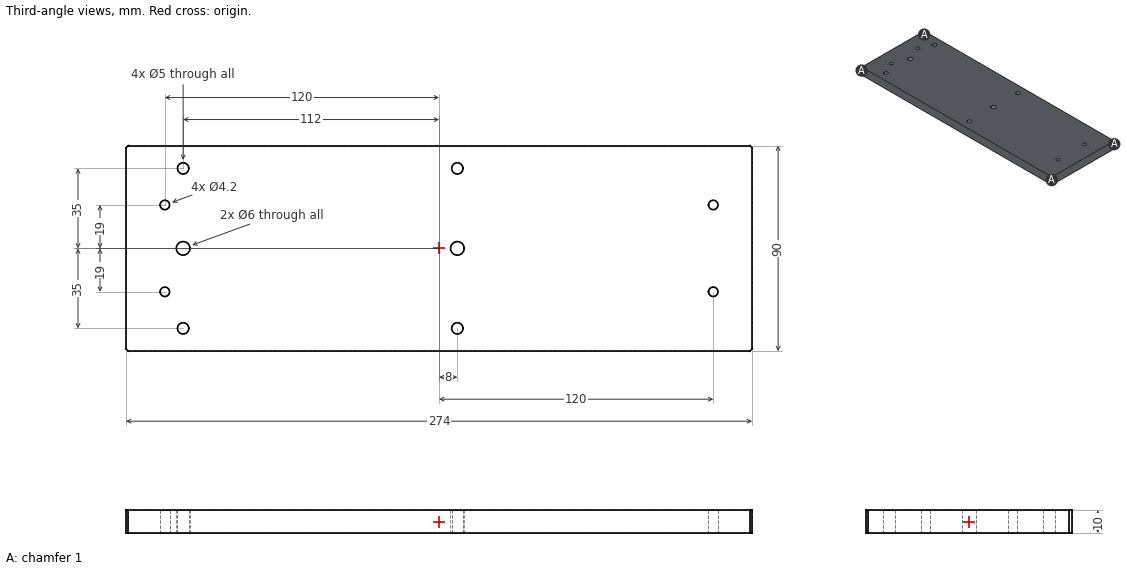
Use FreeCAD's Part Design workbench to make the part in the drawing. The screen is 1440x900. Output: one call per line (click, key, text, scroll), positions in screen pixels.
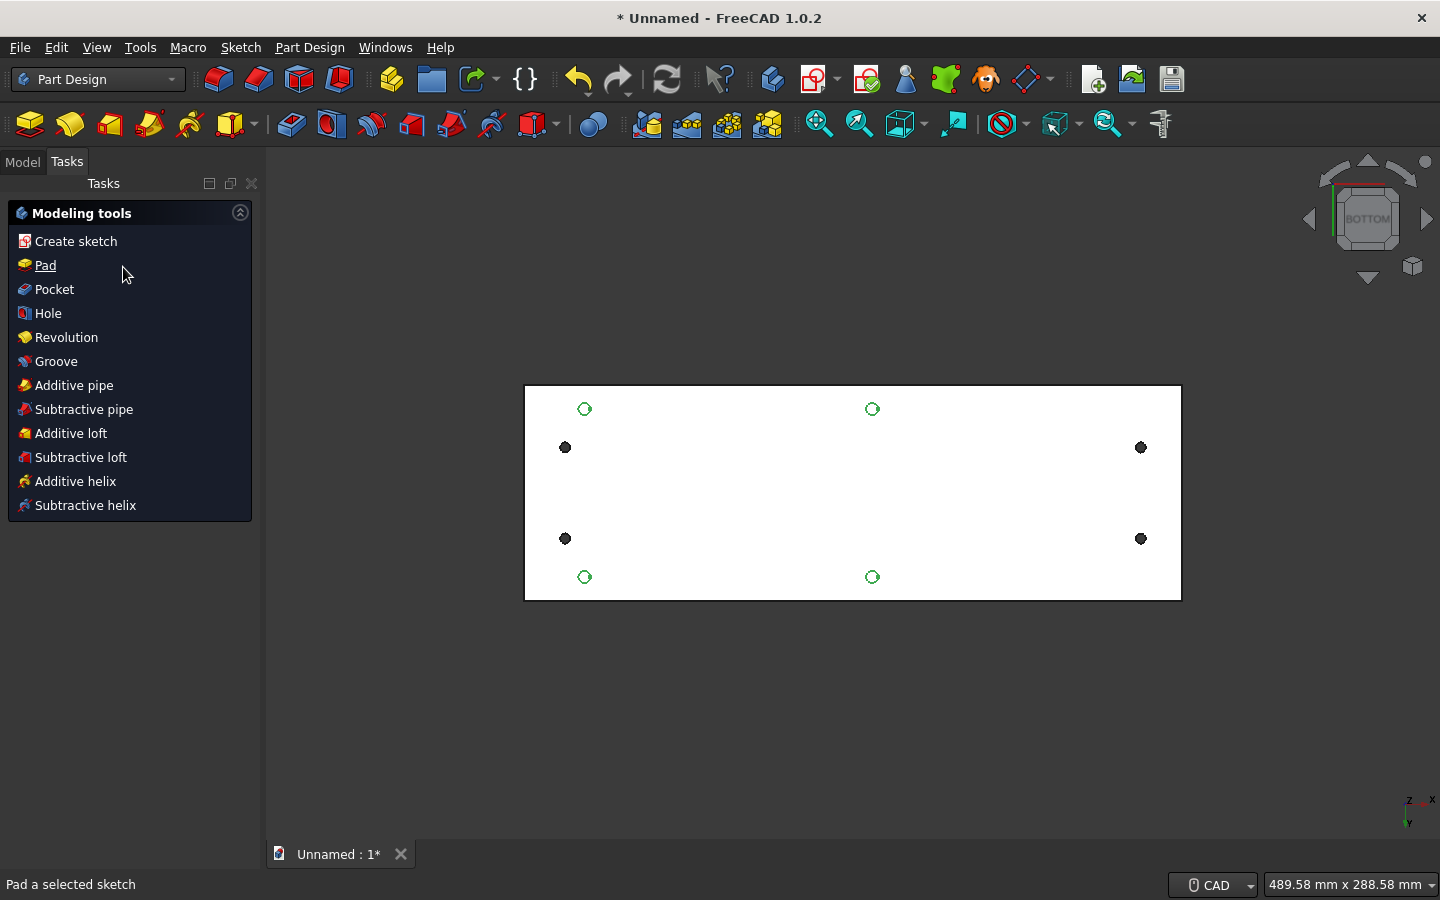
click(332, 124)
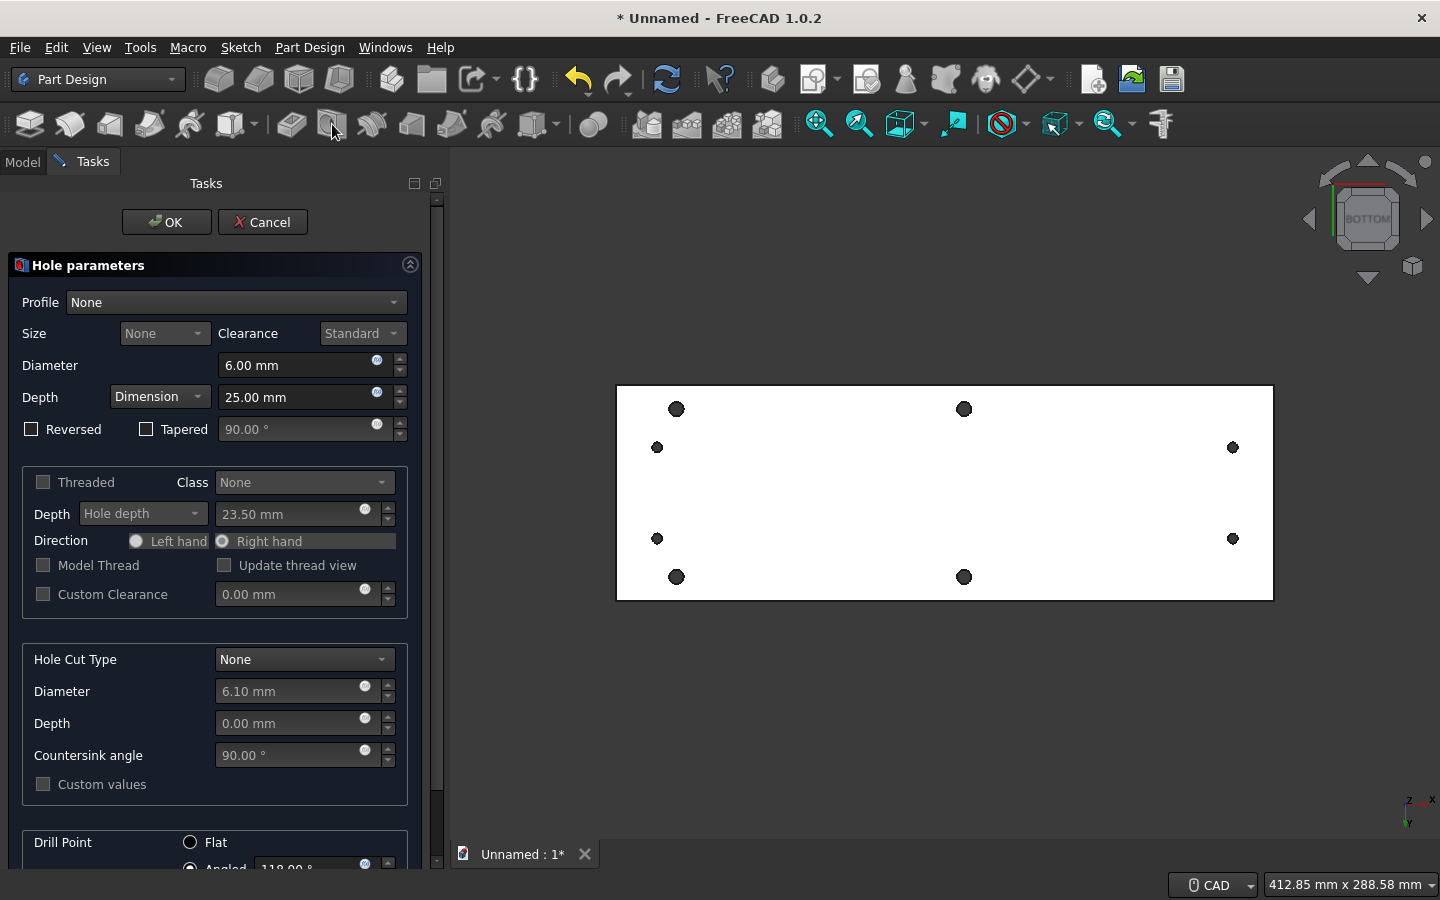
triple_click(305, 365)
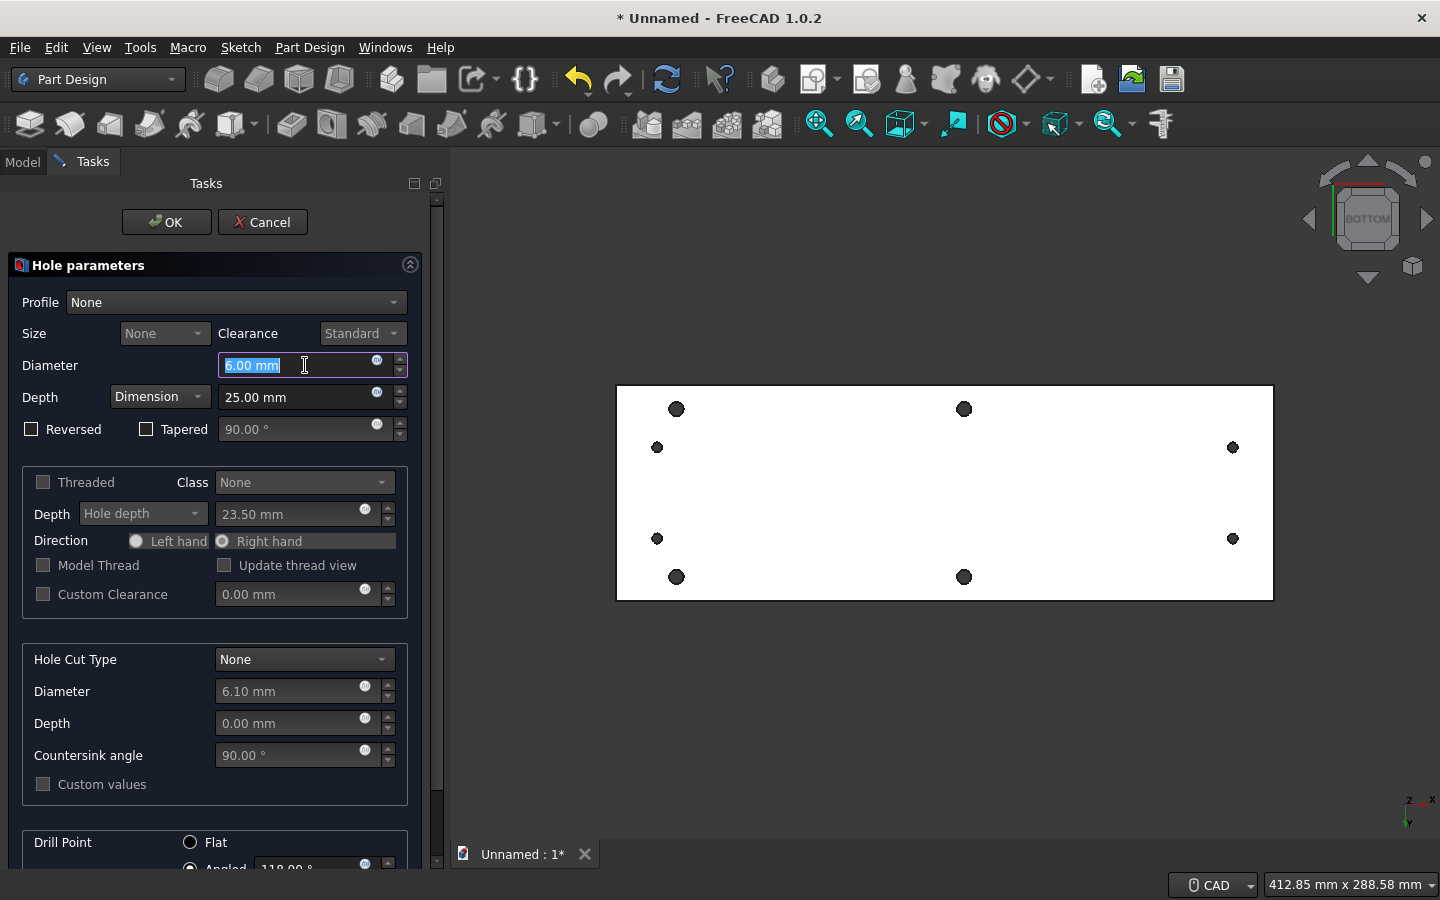
text(5)
key(Tab)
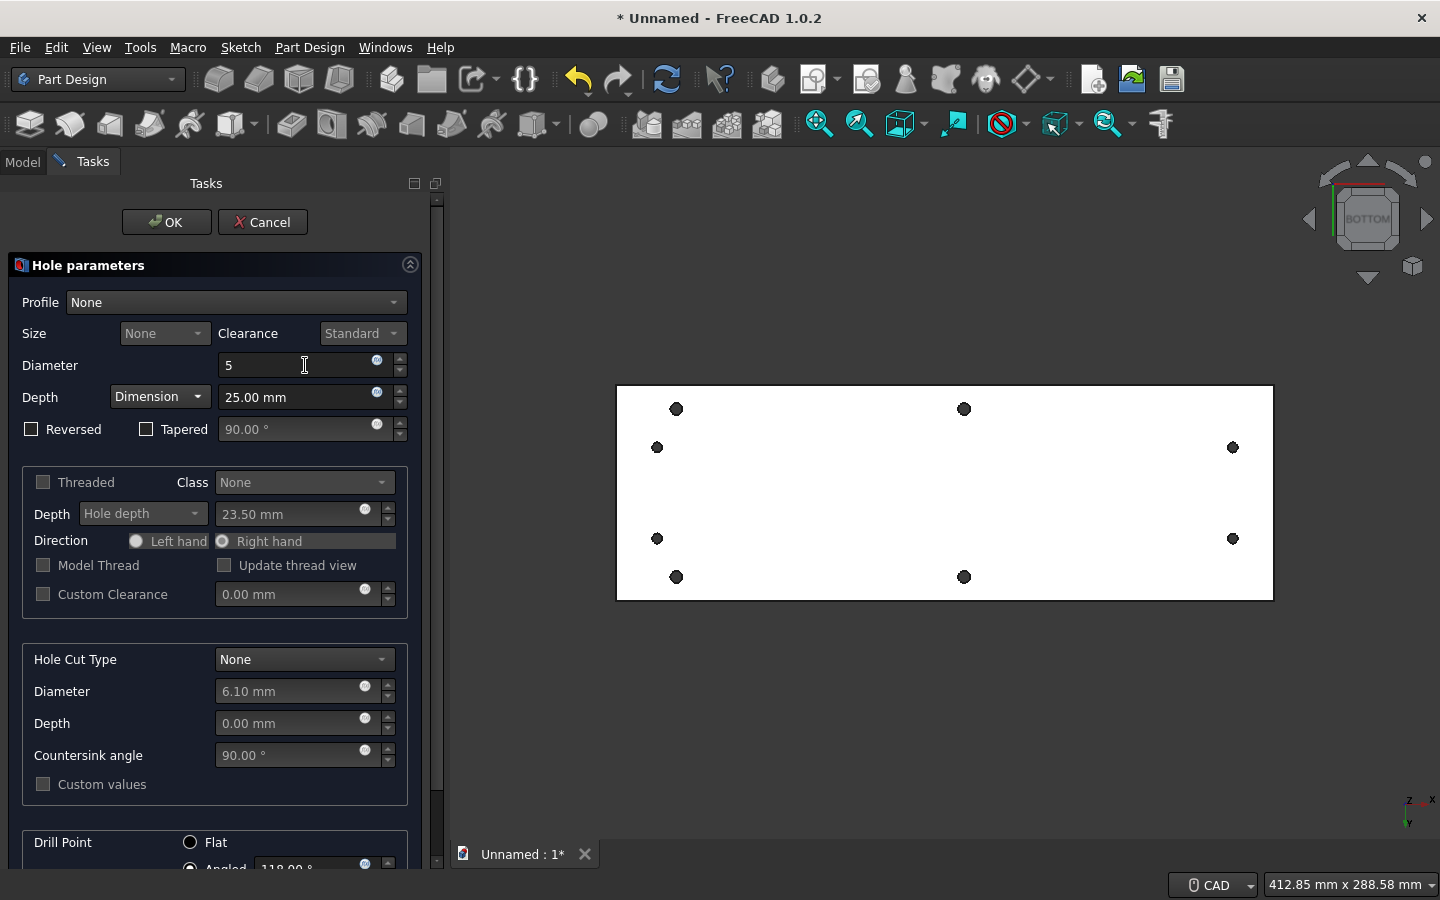
click(161, 396)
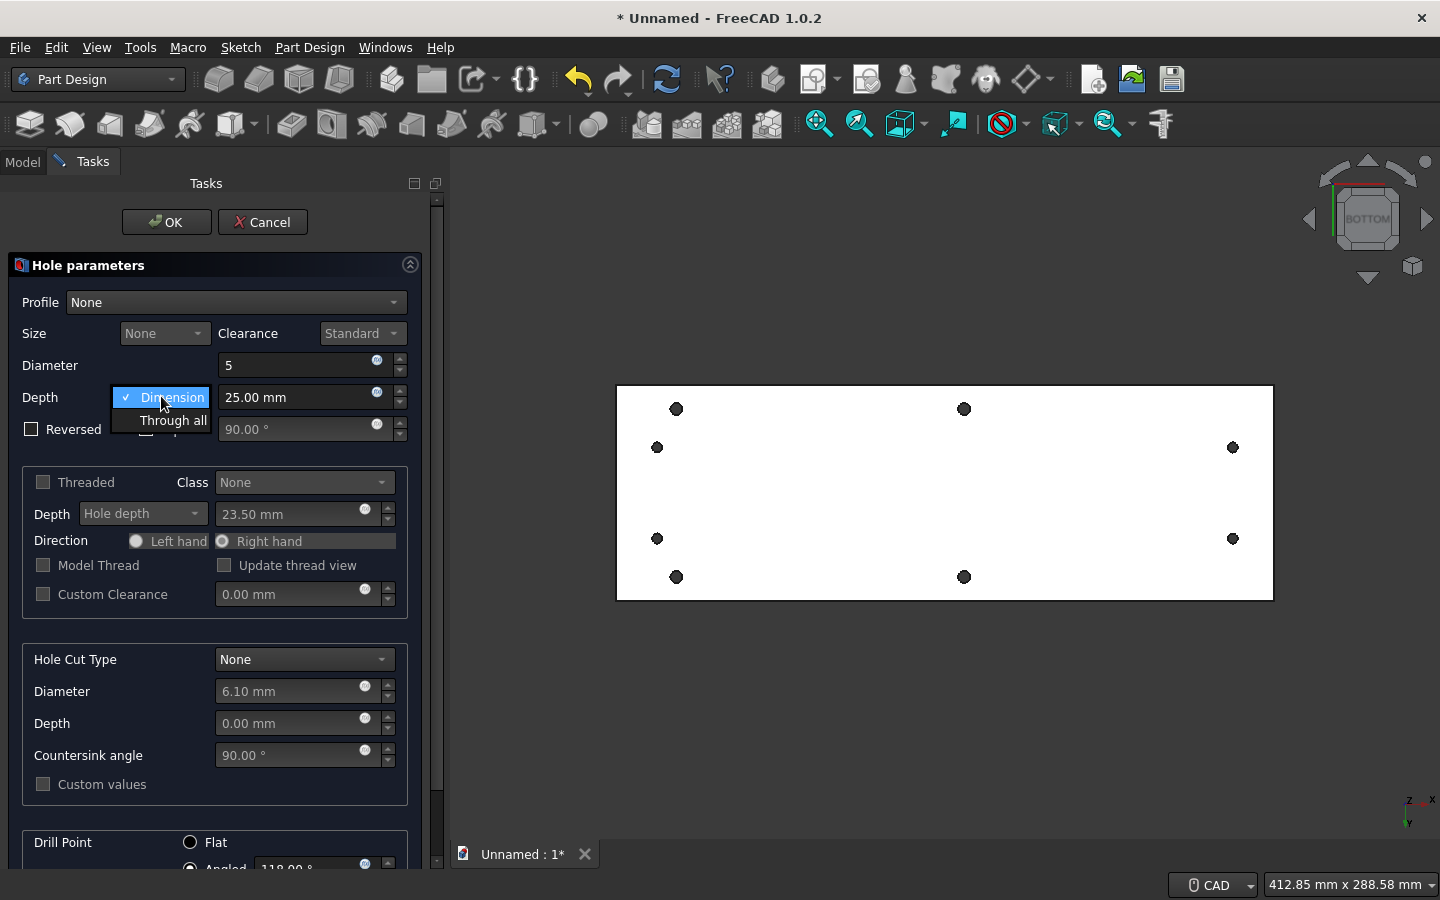
click(160, 420)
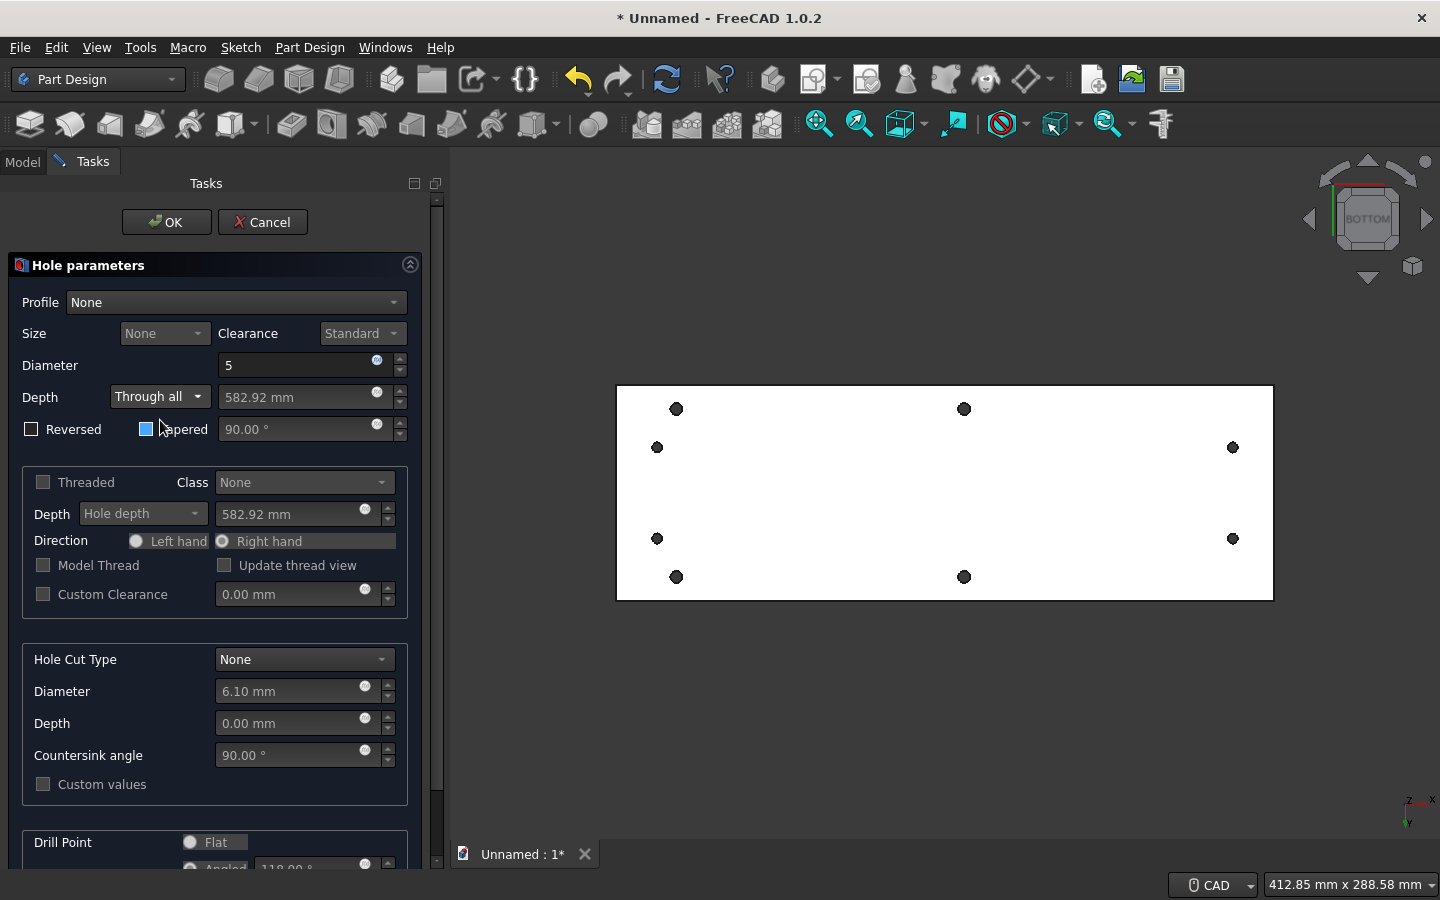
click(167, 222)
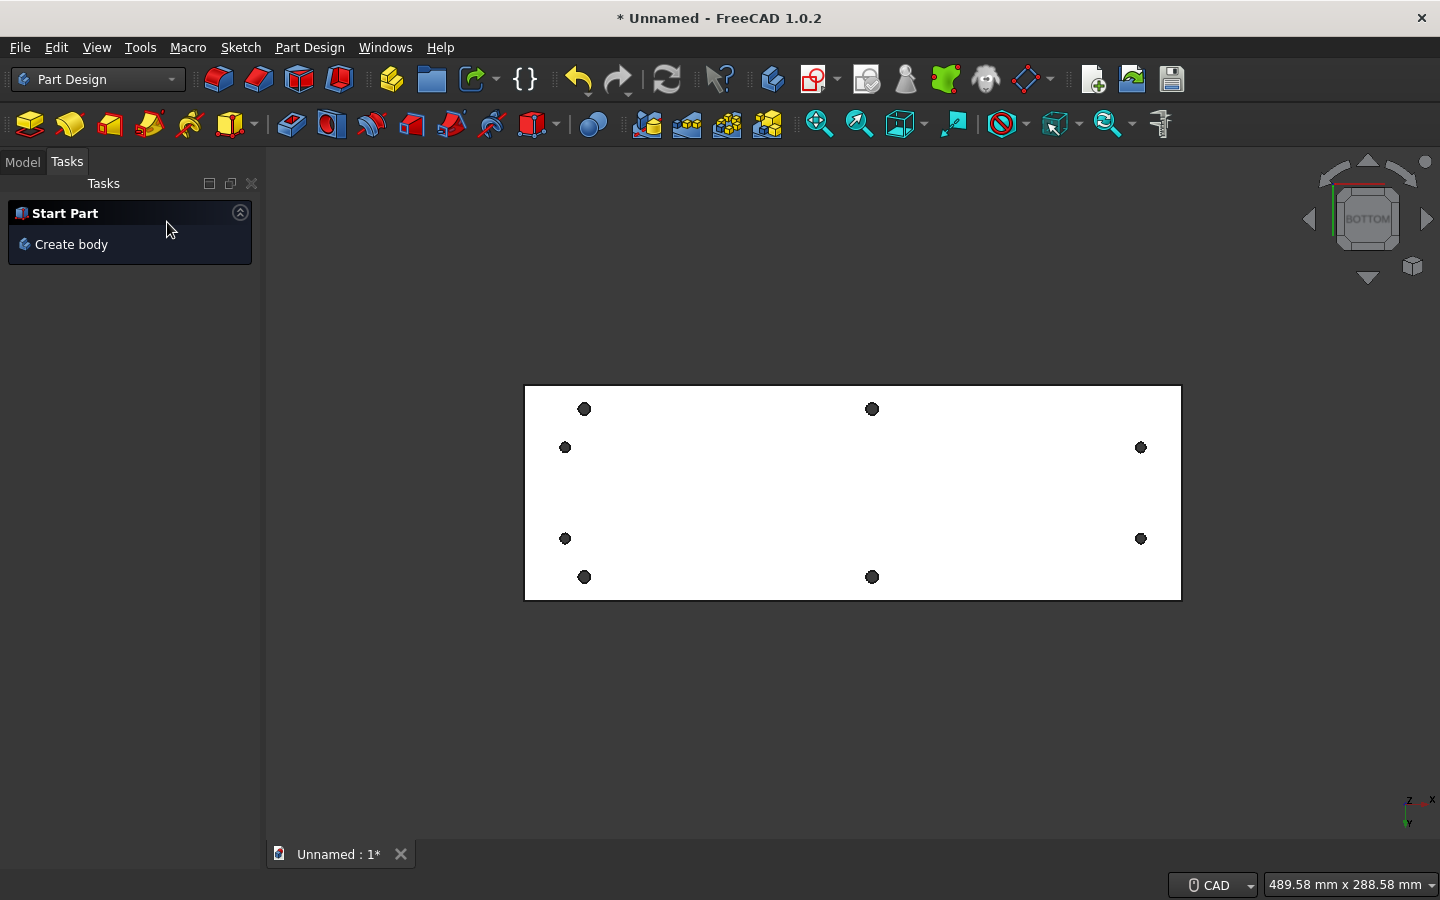
click(759, 492)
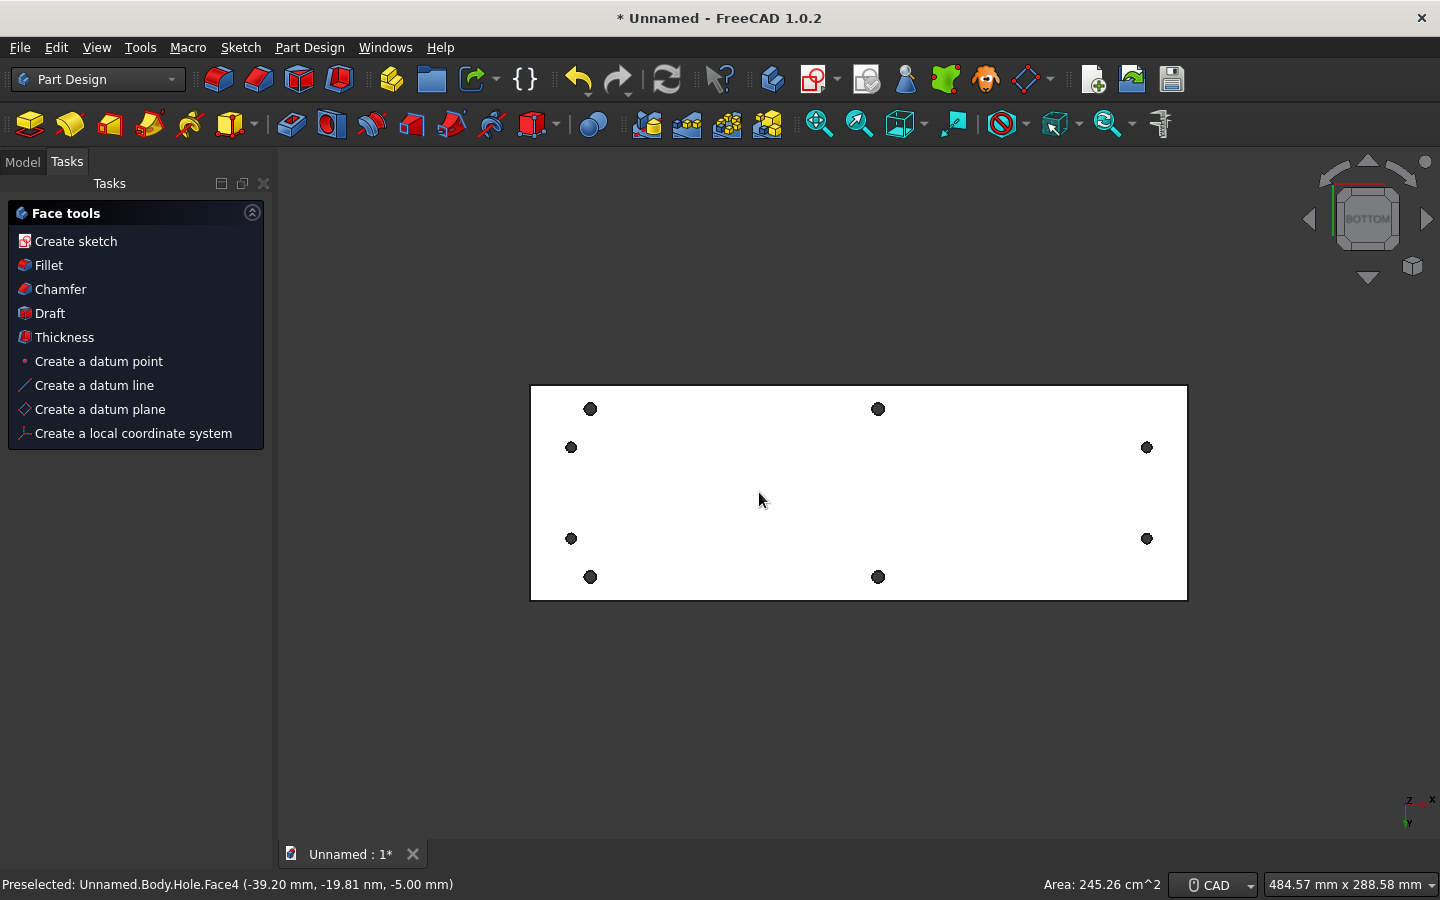
click(814, 80)